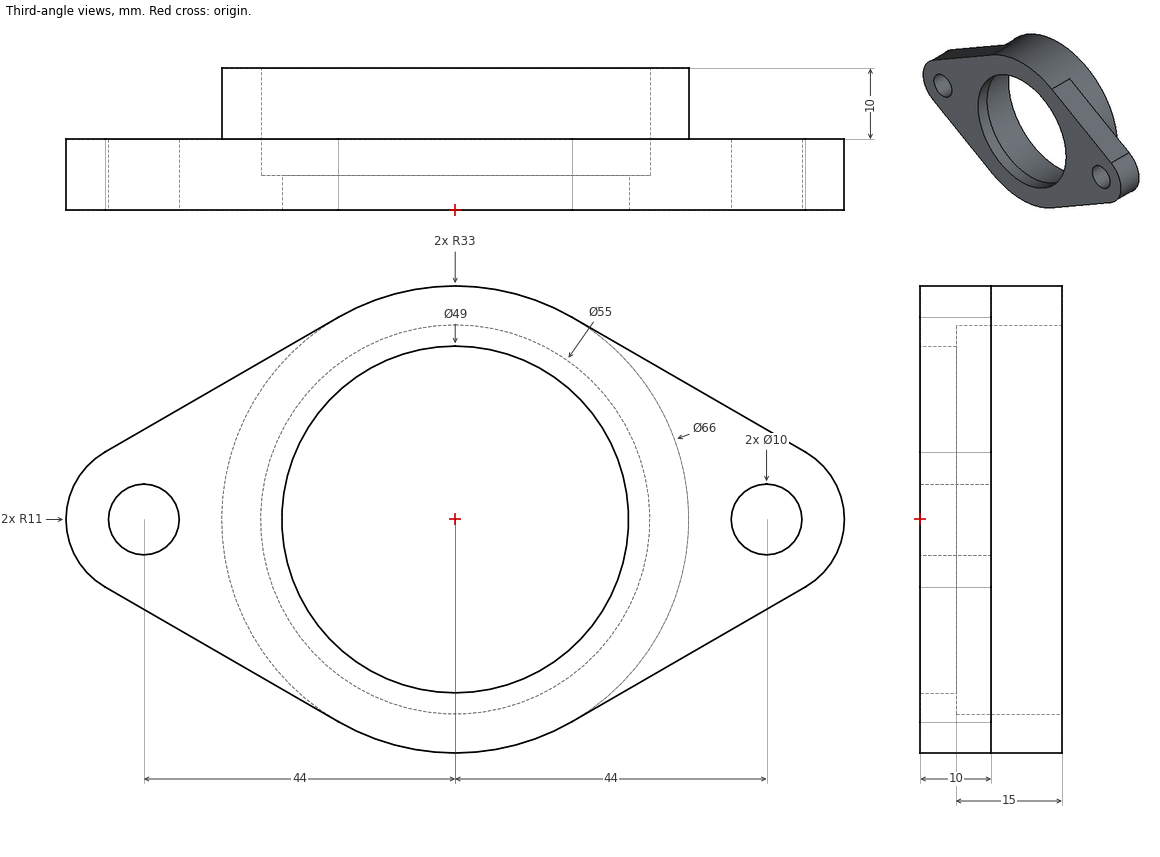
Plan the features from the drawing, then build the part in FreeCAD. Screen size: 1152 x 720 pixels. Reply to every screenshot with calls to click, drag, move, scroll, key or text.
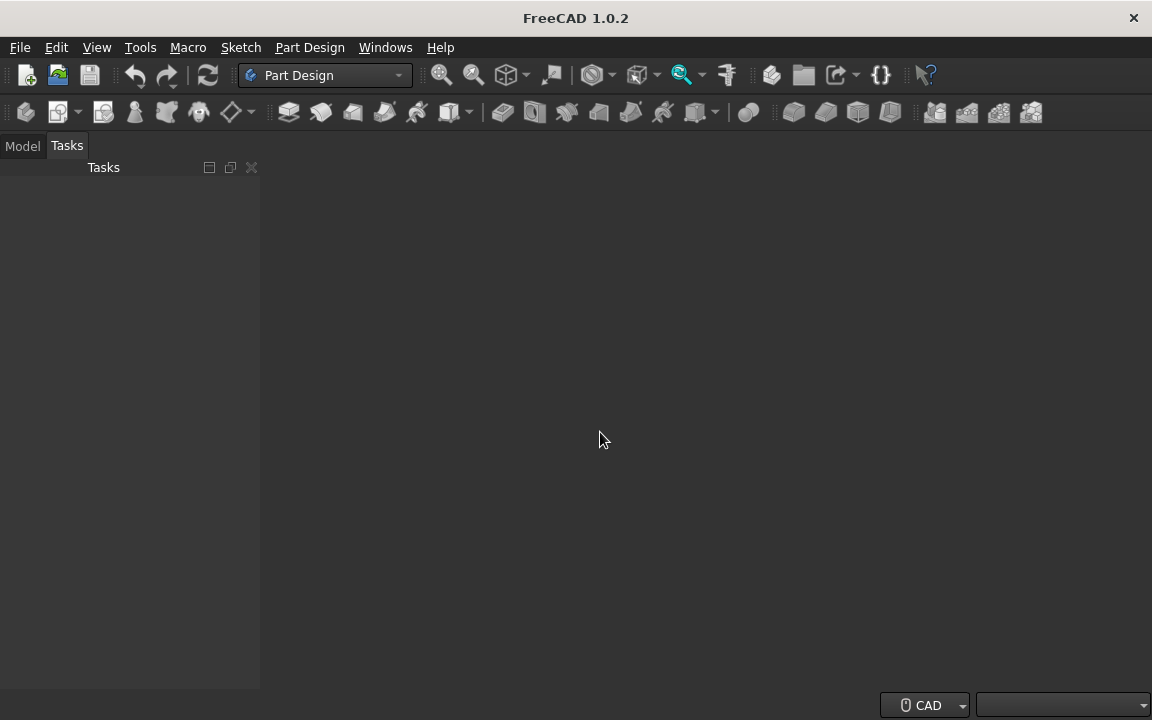
click(26, 76)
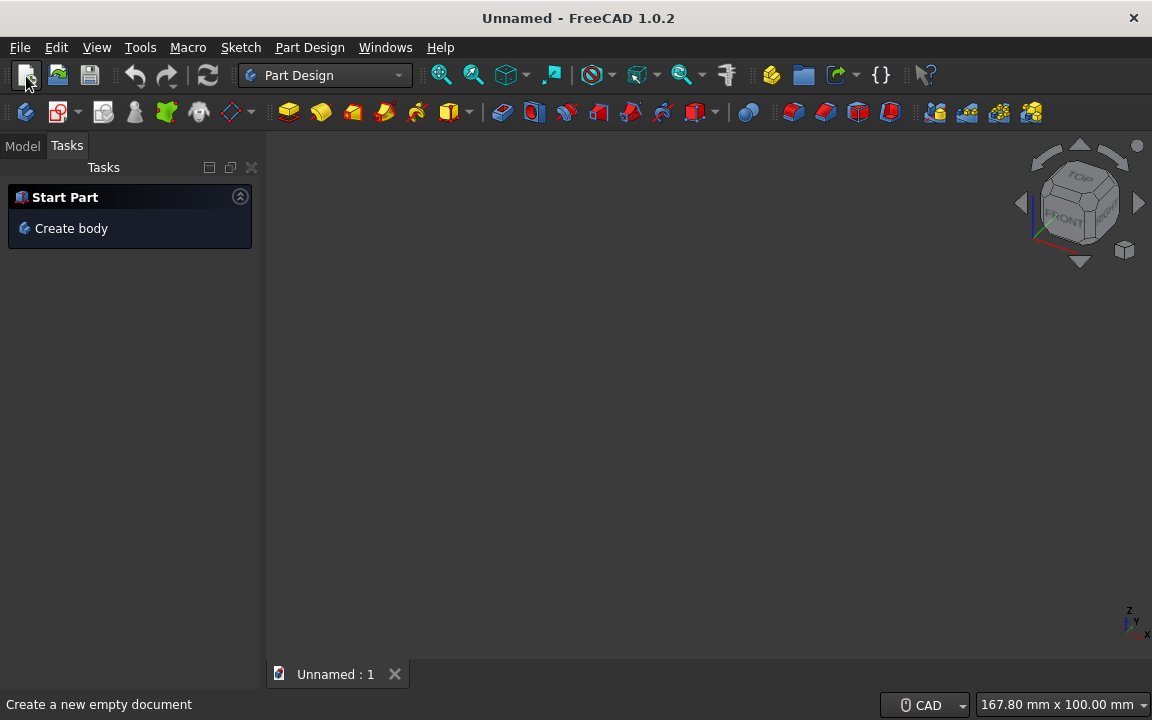
click(58, 112)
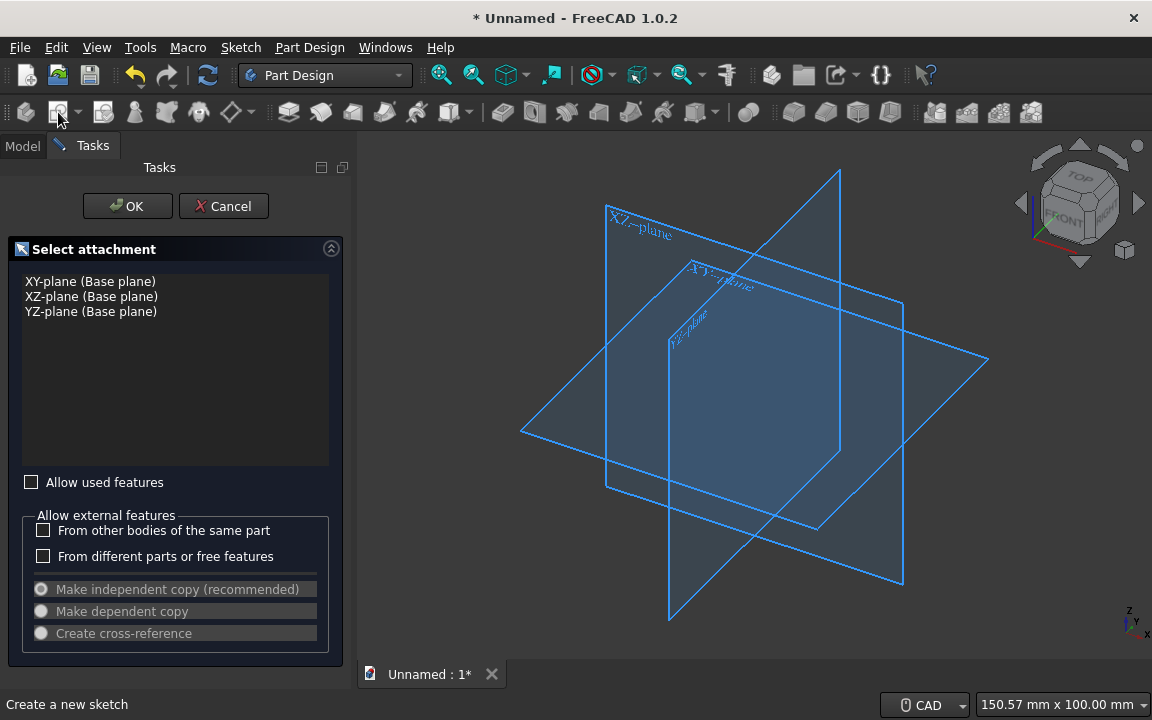
click(82, 296)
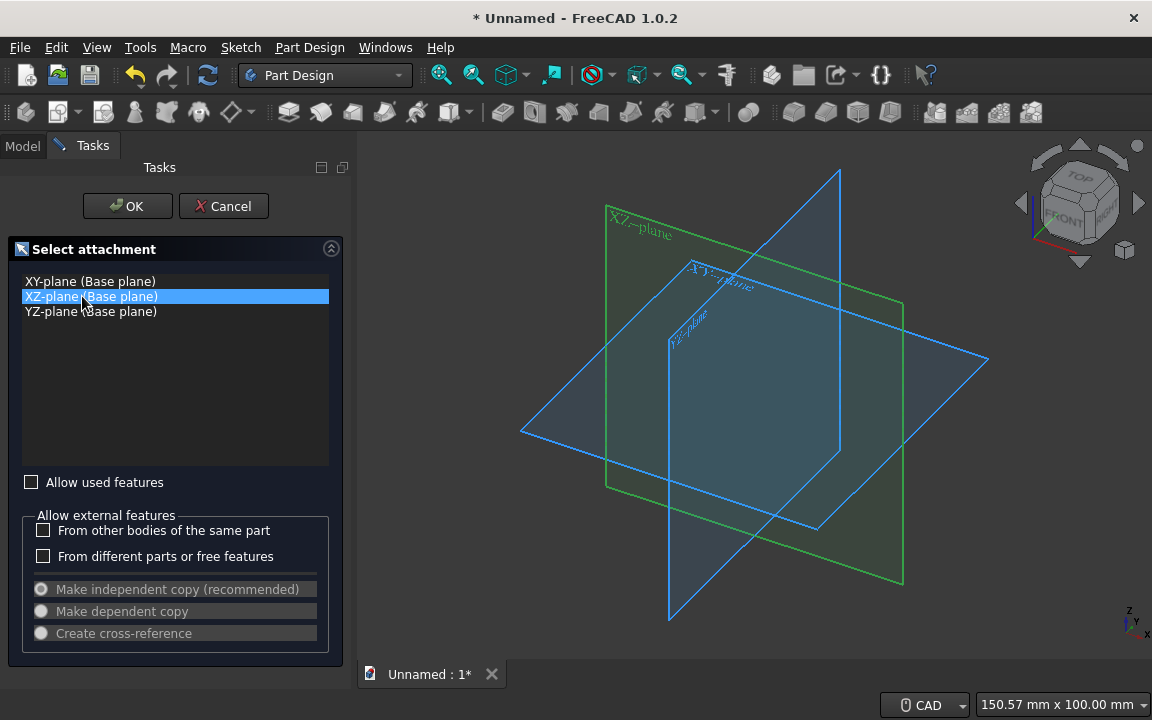
click(128, 206)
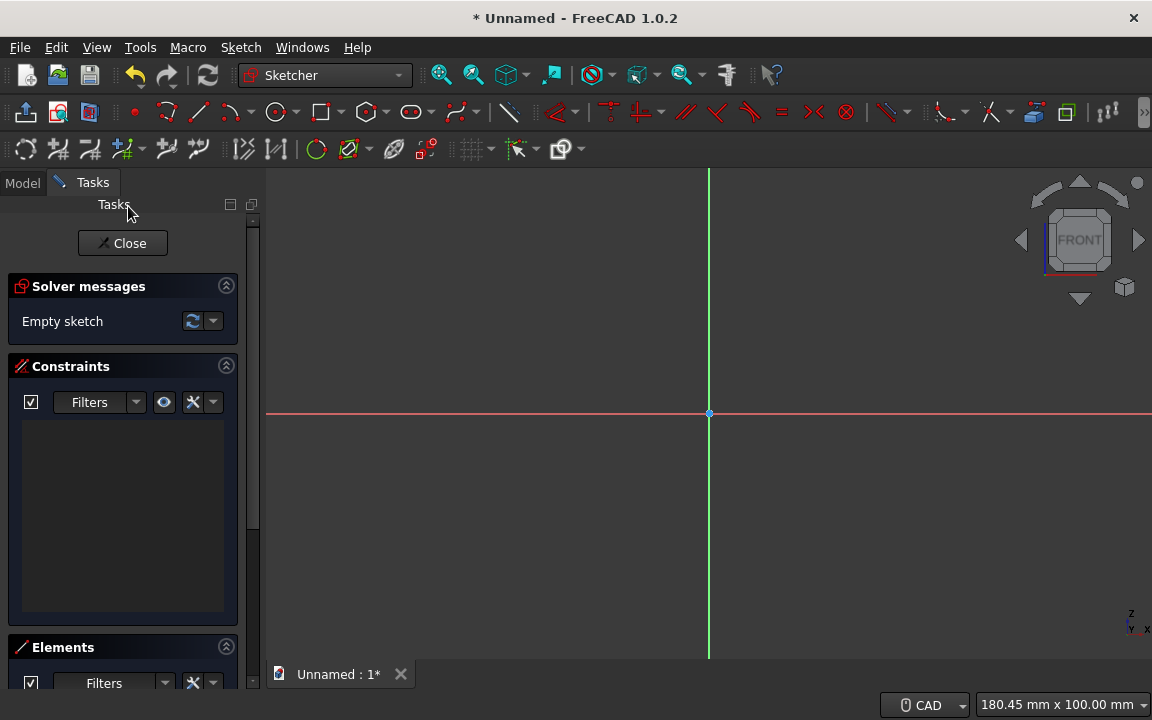
scroll(331, 413, down, 1)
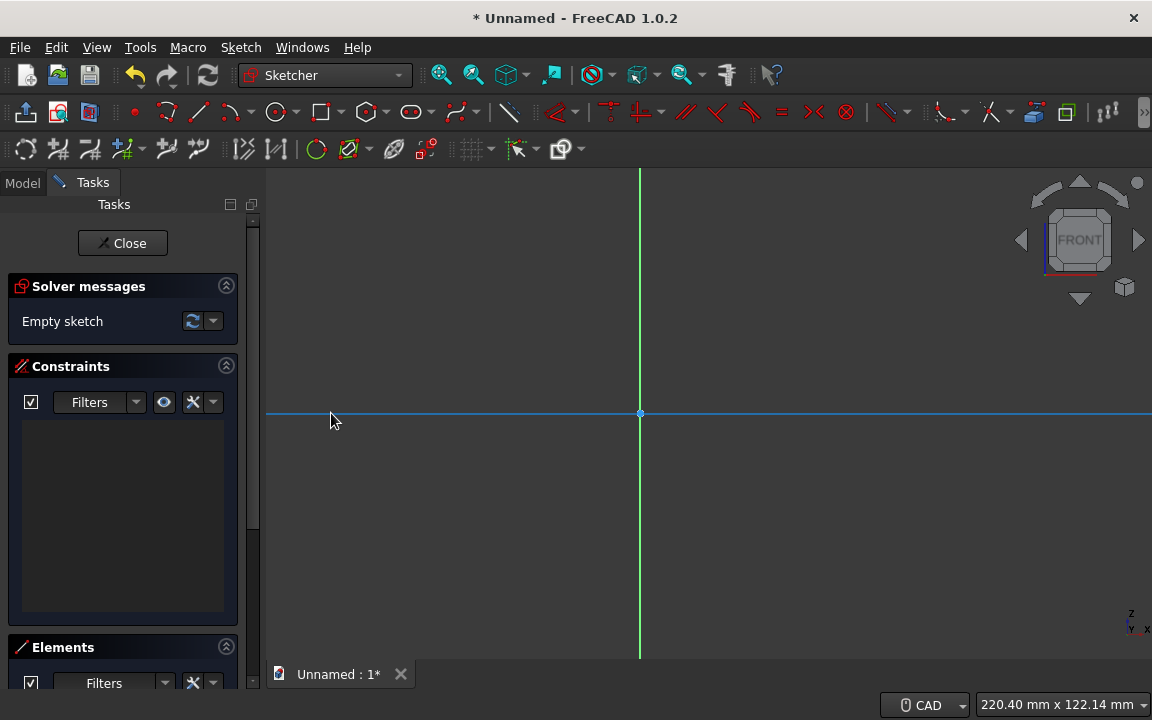
click(200, 112)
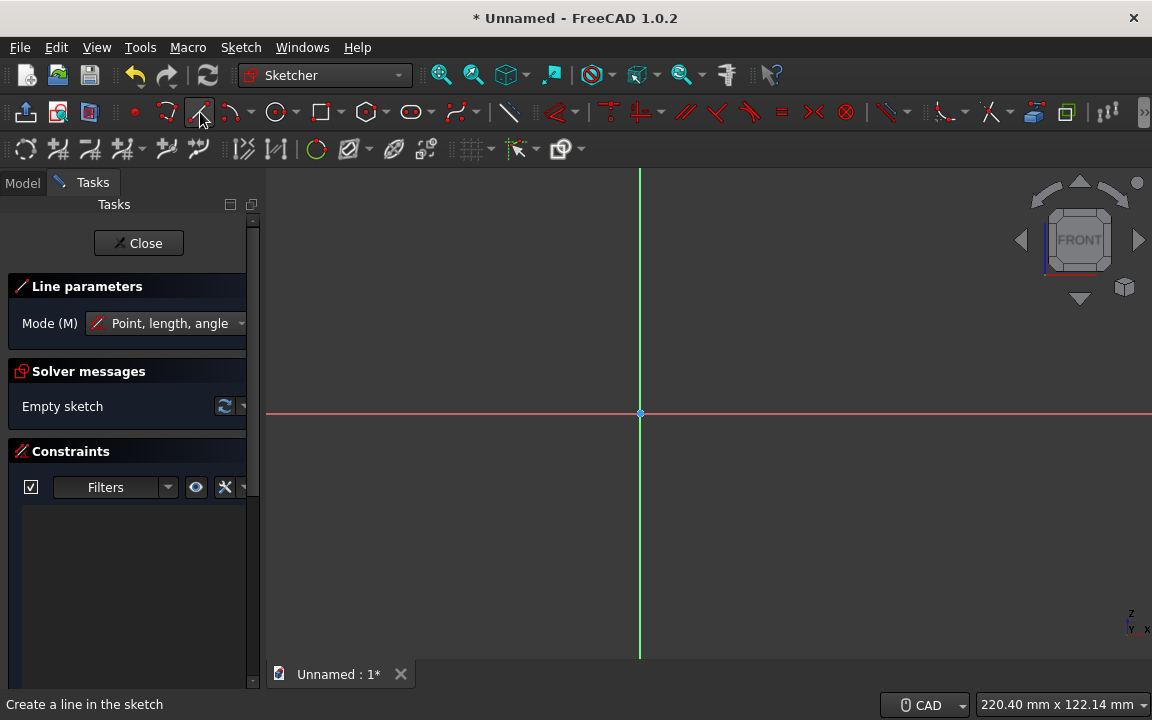
click(574, 528)
click(442, 452)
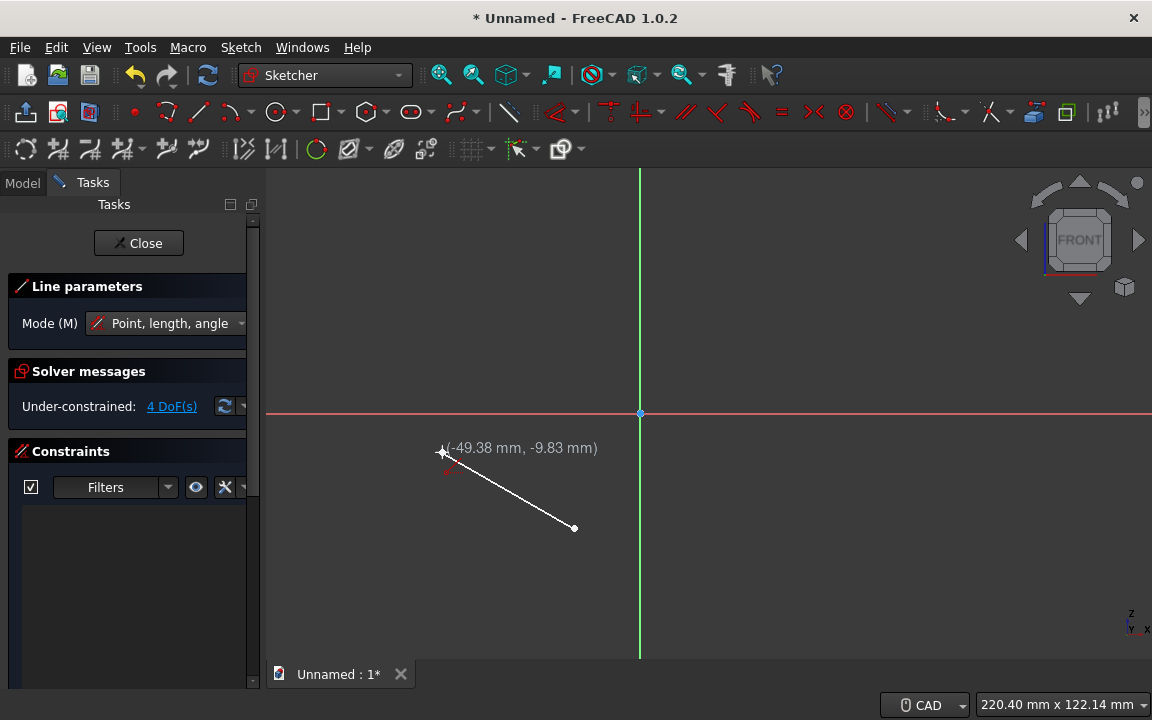
click(442, 375)
click(574, 299)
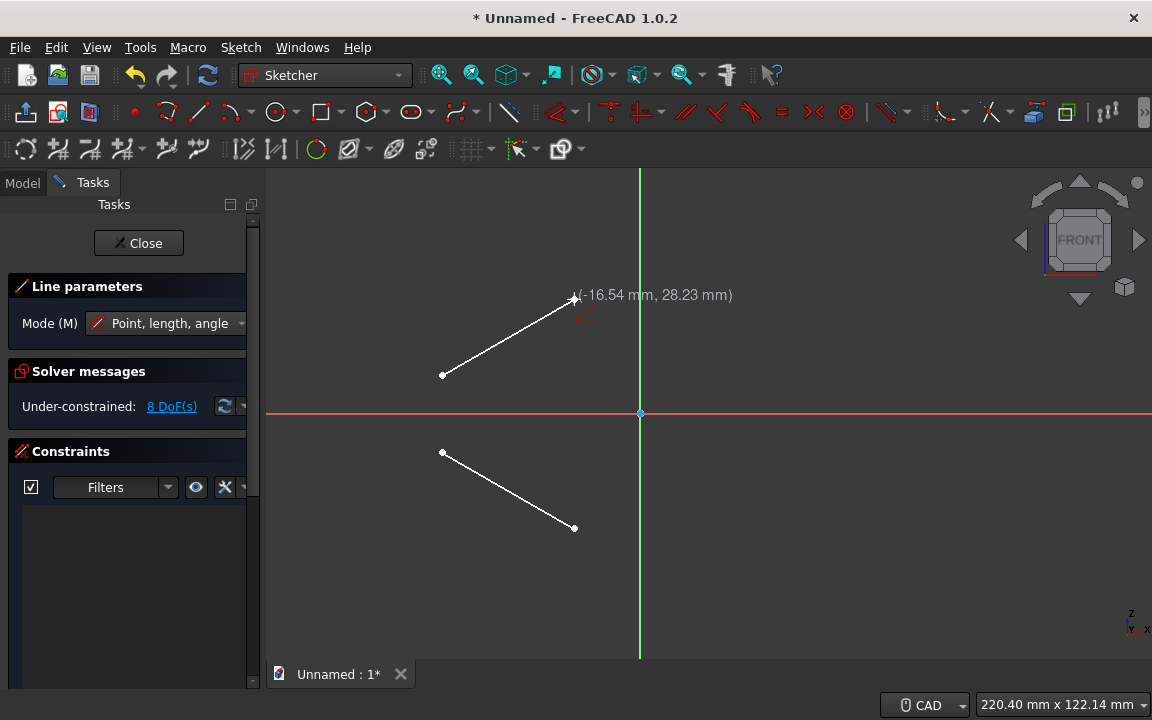
click(707, 299)
click(839, 375)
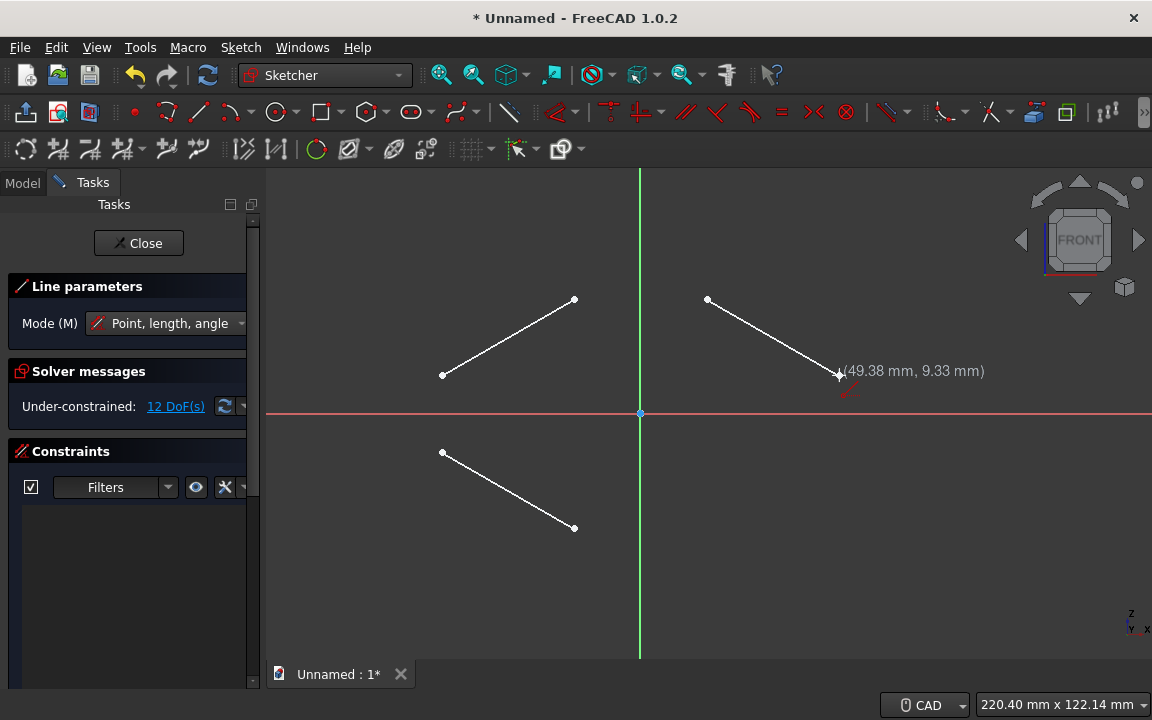
click(839, 452)
click(707, 528)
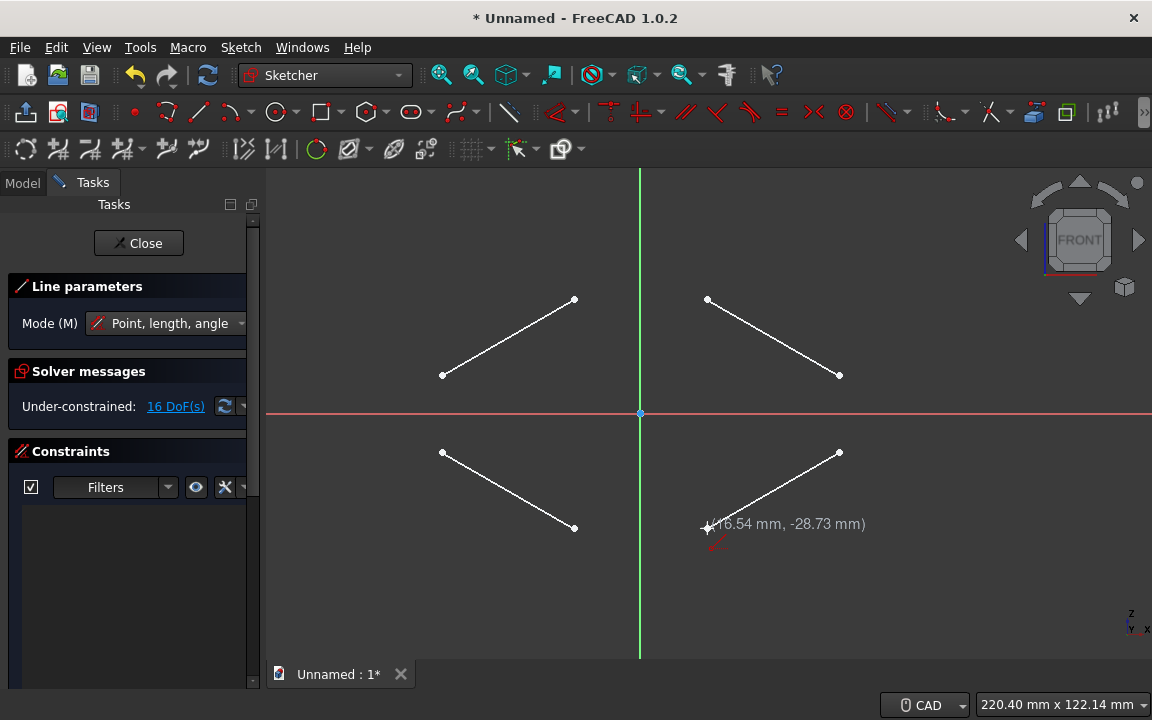
click(254, 112)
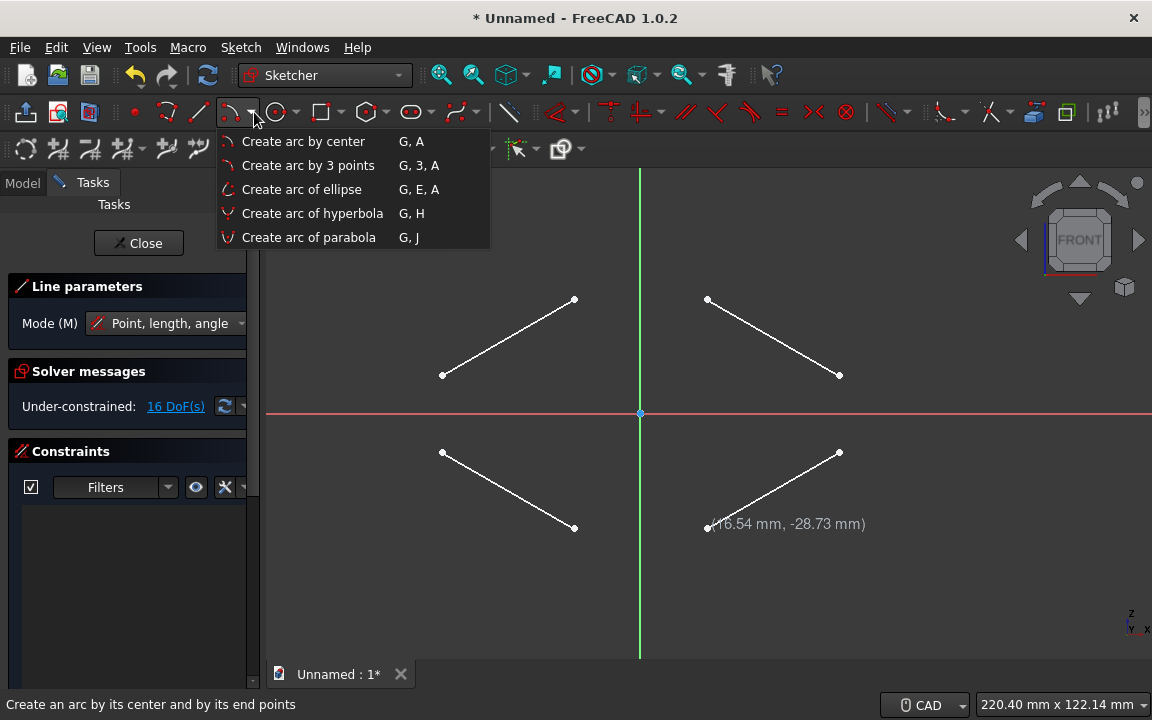
click(354, 165)